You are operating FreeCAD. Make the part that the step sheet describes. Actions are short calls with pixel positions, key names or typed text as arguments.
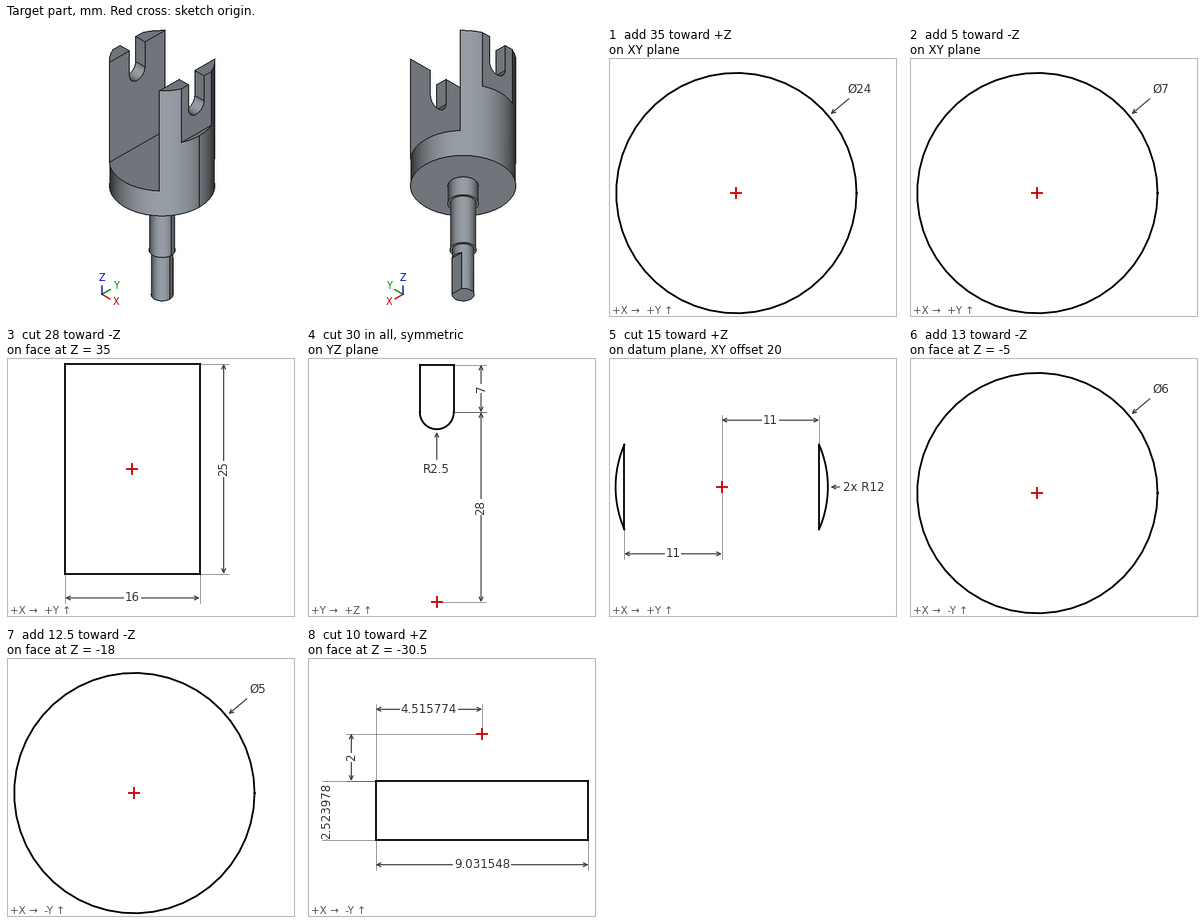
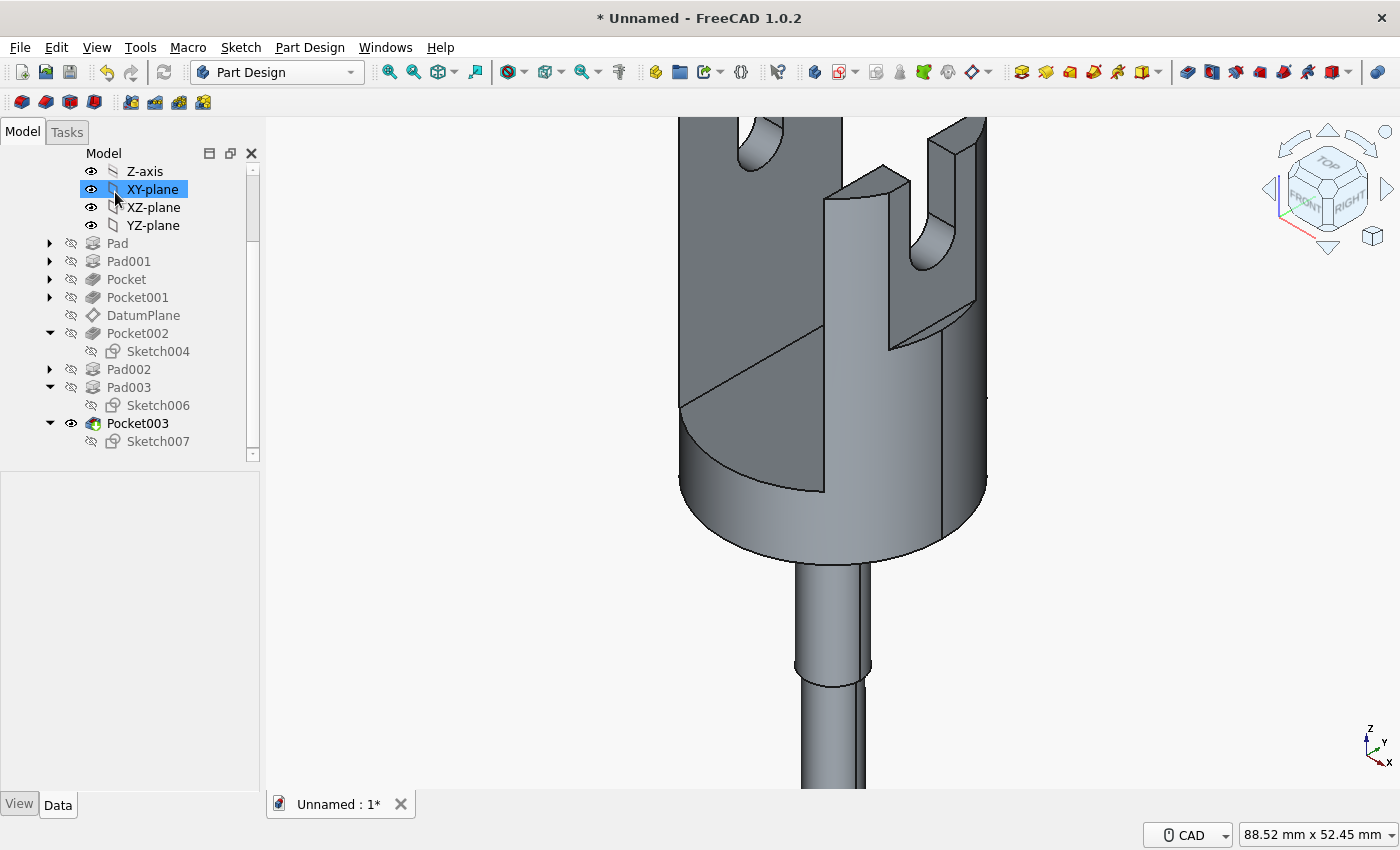
click(390, 72)